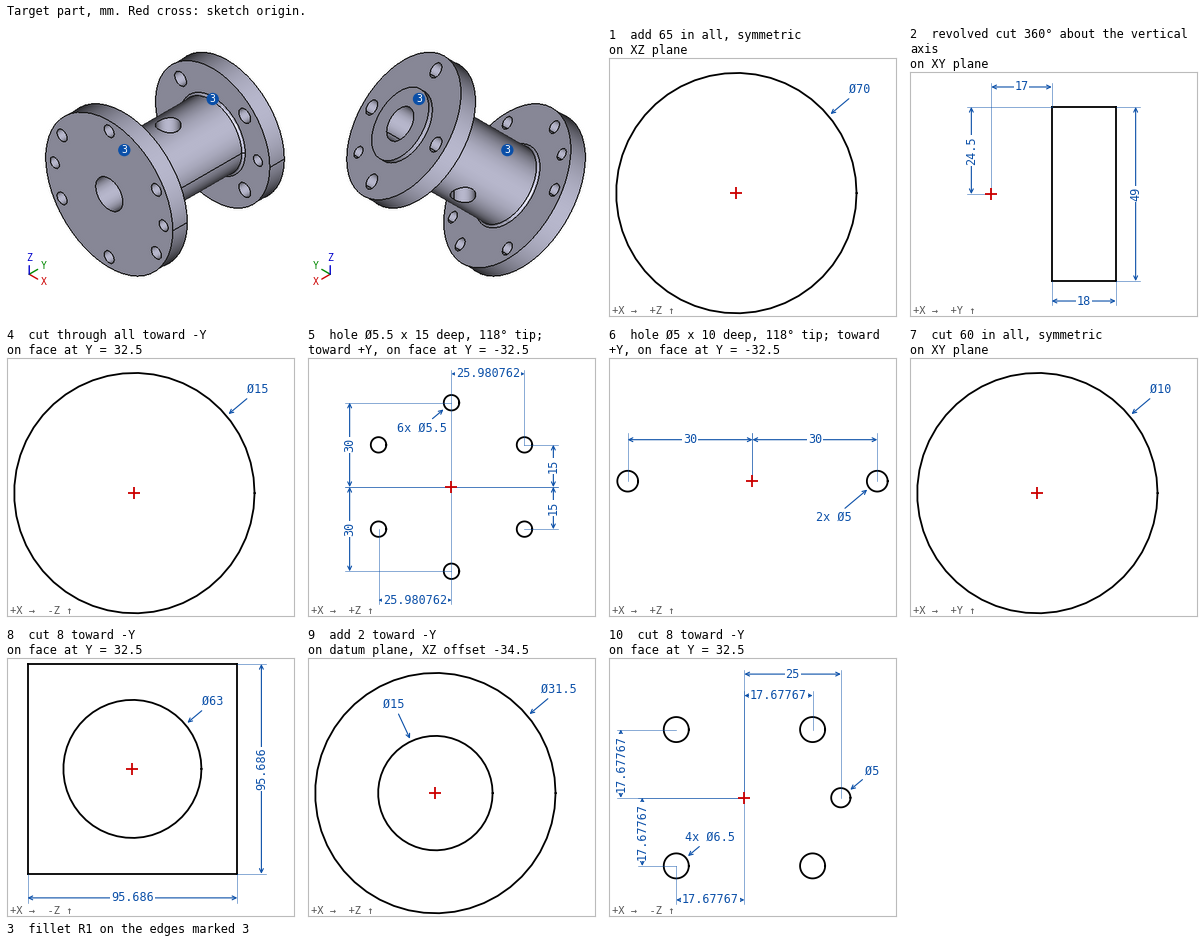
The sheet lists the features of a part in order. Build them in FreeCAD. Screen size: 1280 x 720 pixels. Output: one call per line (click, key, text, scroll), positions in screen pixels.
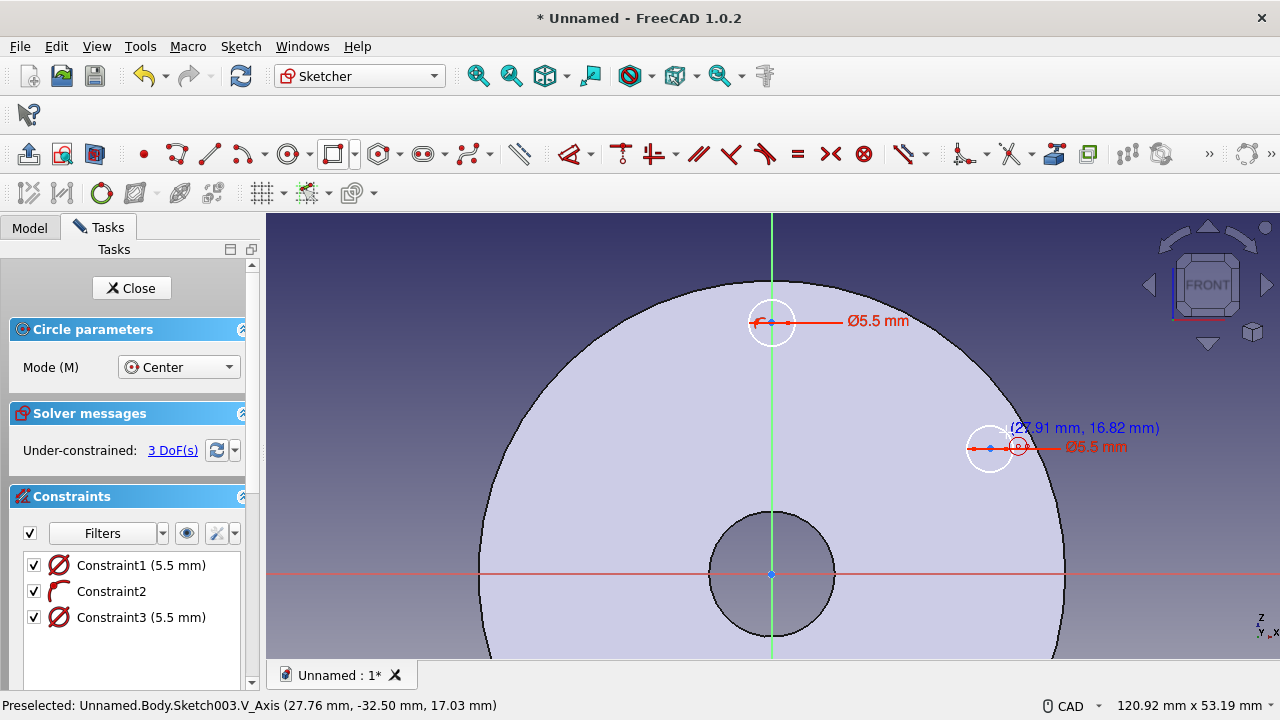
scroll(622, 268, down, 3)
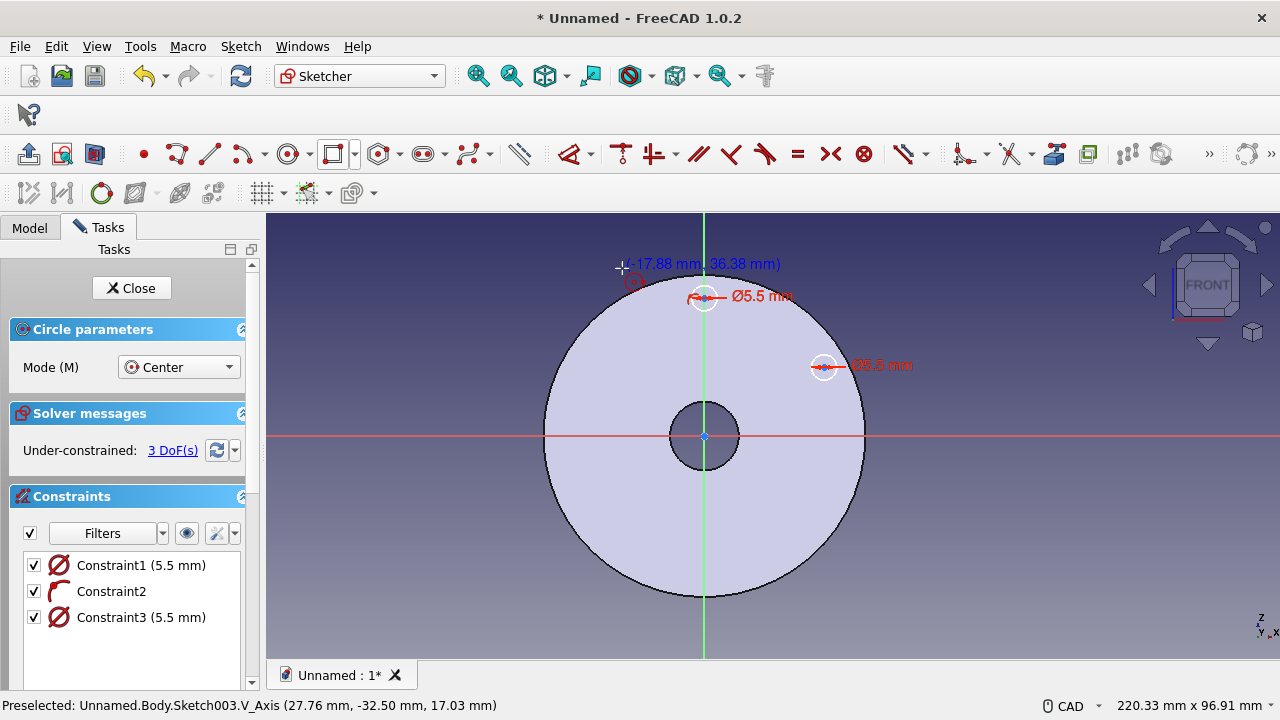
scroll(824, 505, up, 3)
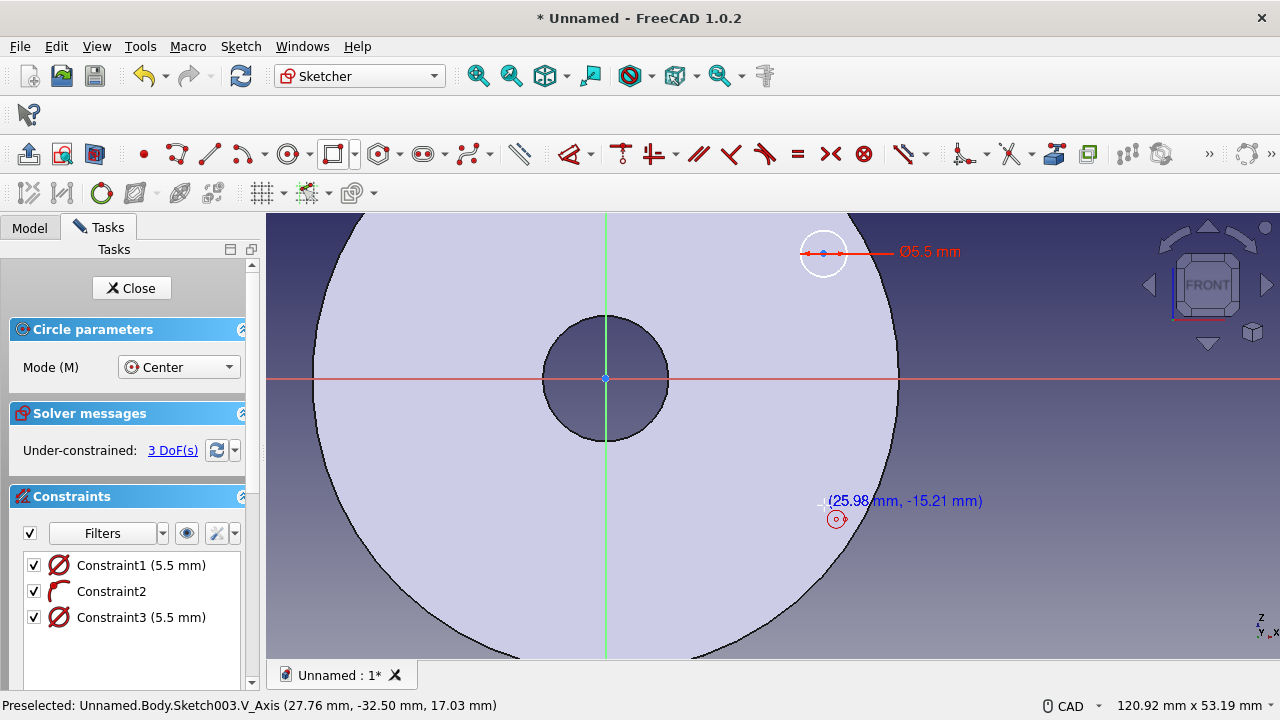
click(824, 505)
move(840, 488)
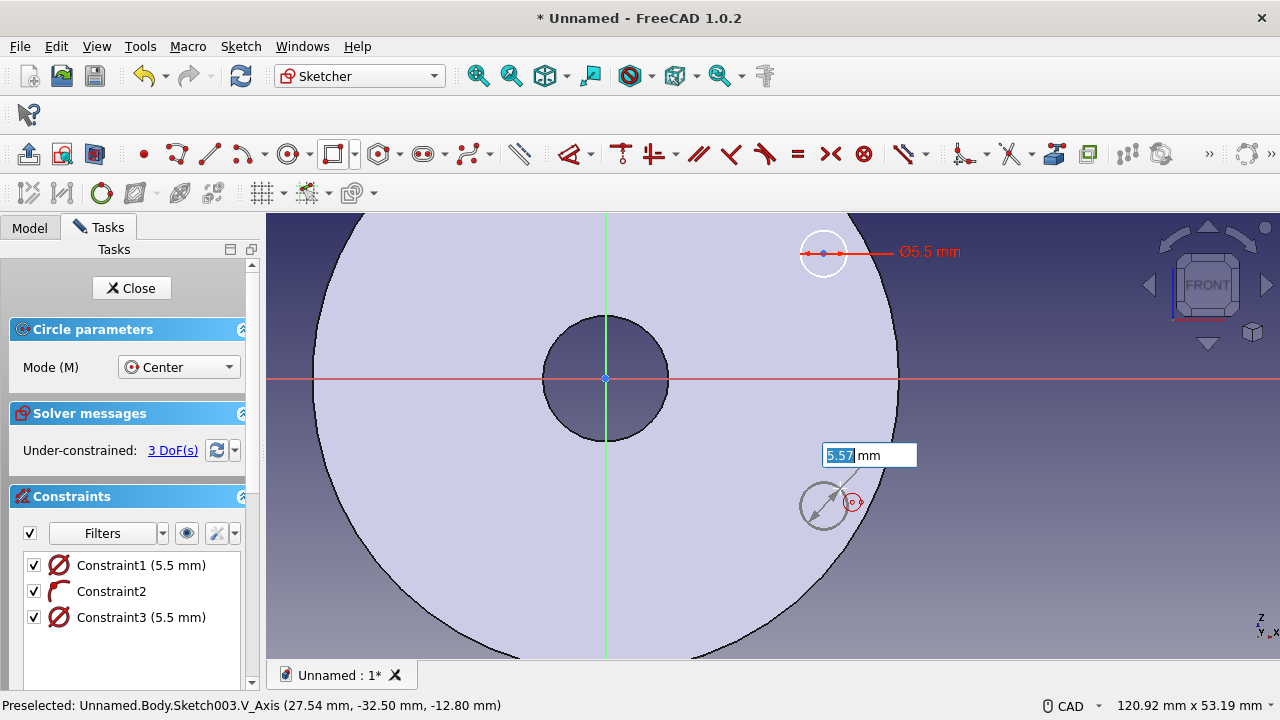
text(5.5)
key(Return)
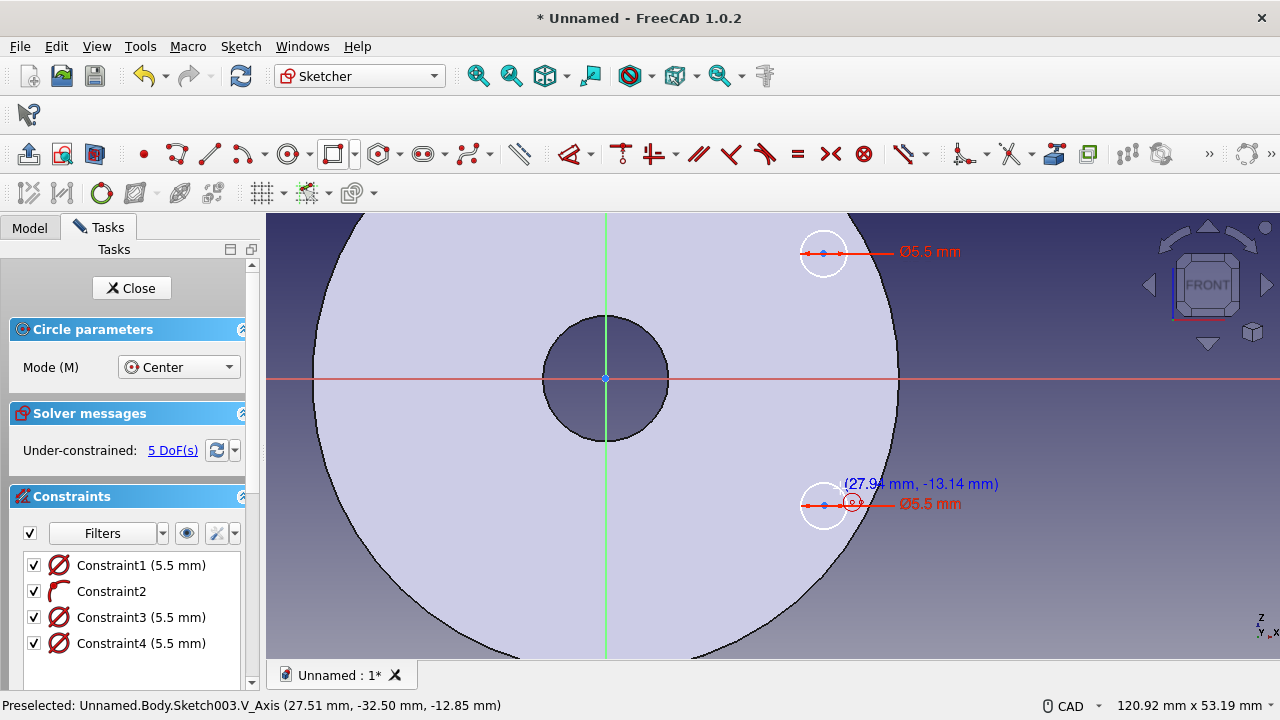
click(606, 630)
move(622, 614)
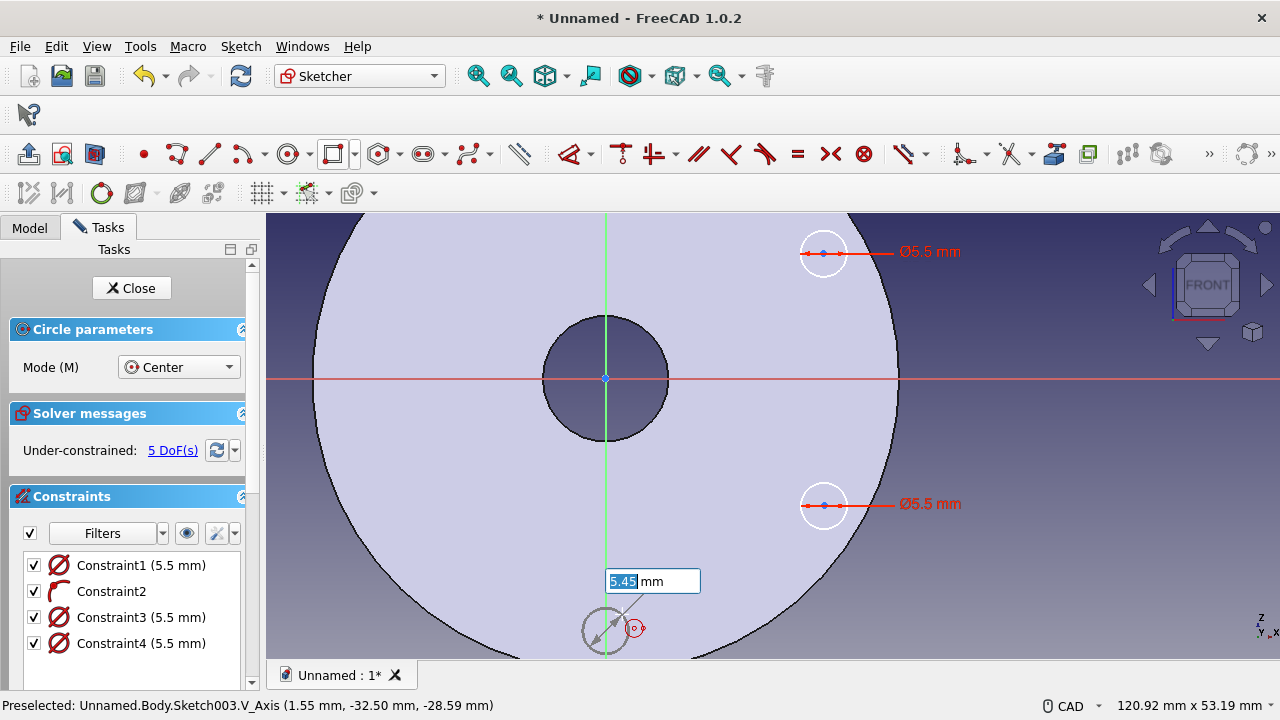
text(5.5)
key(Return)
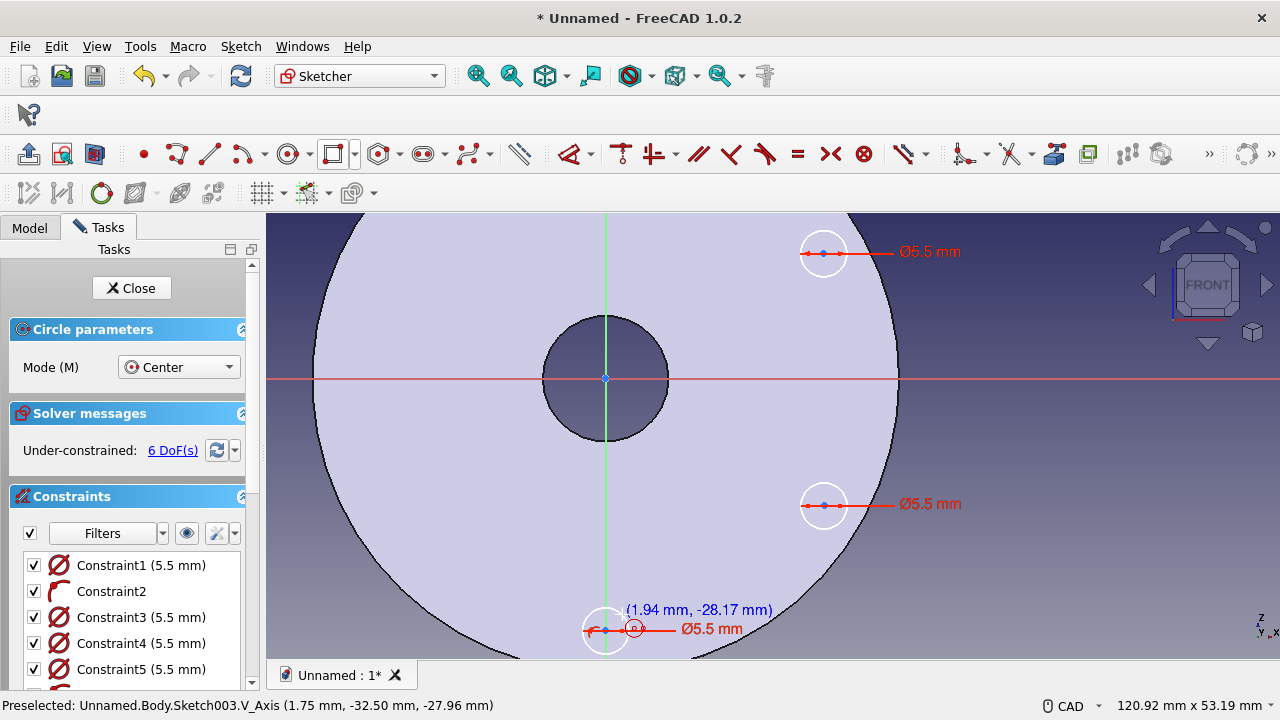
click(388, 505)
move(404, 488)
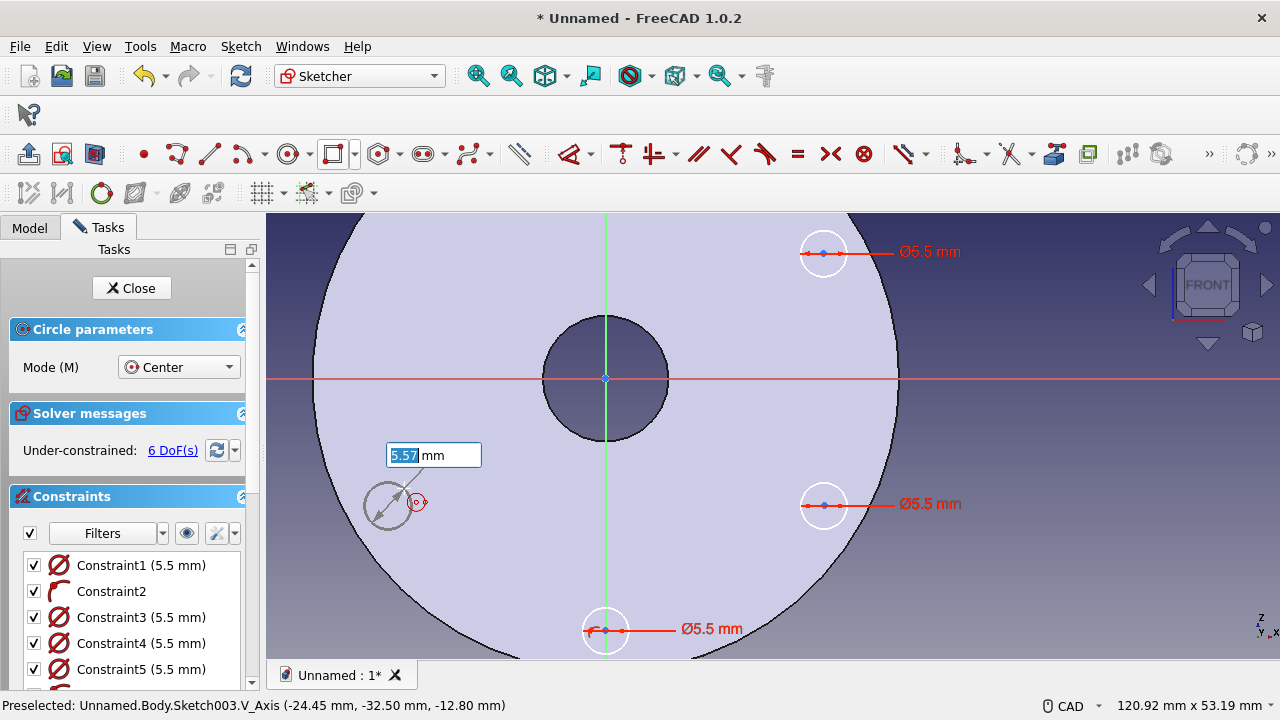
text(5.5)
key(Return)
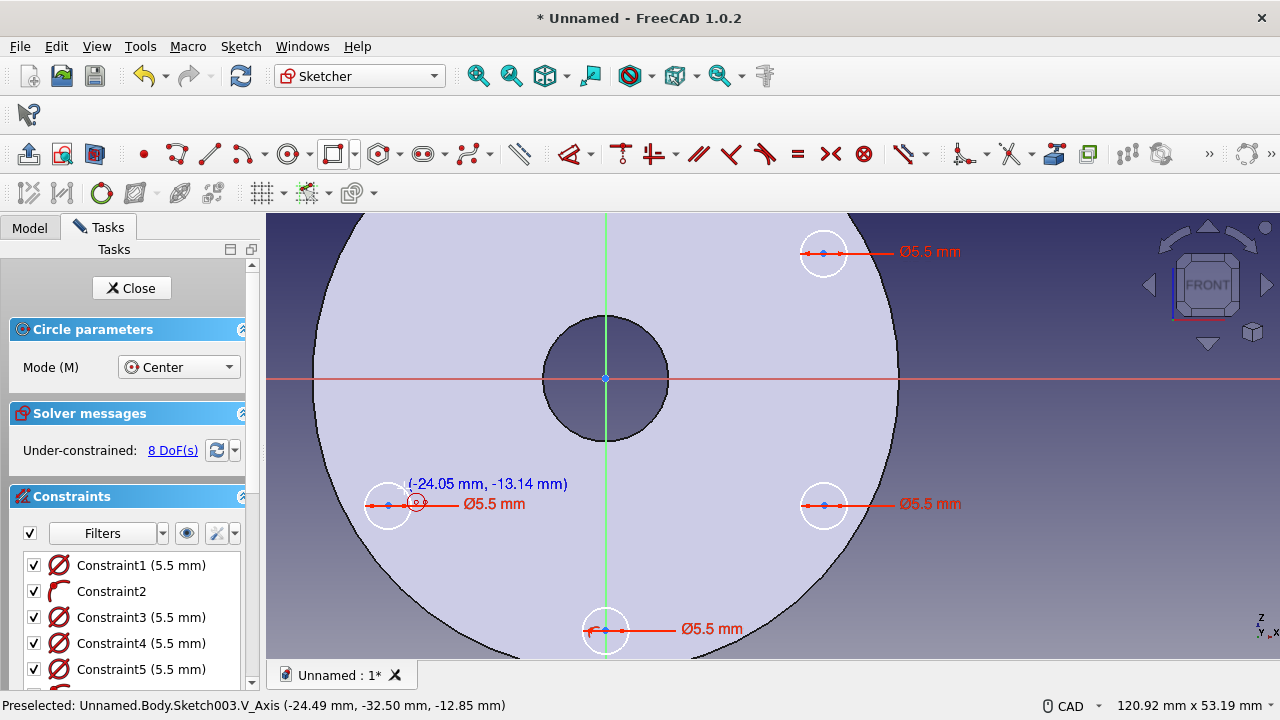
click(388, 253)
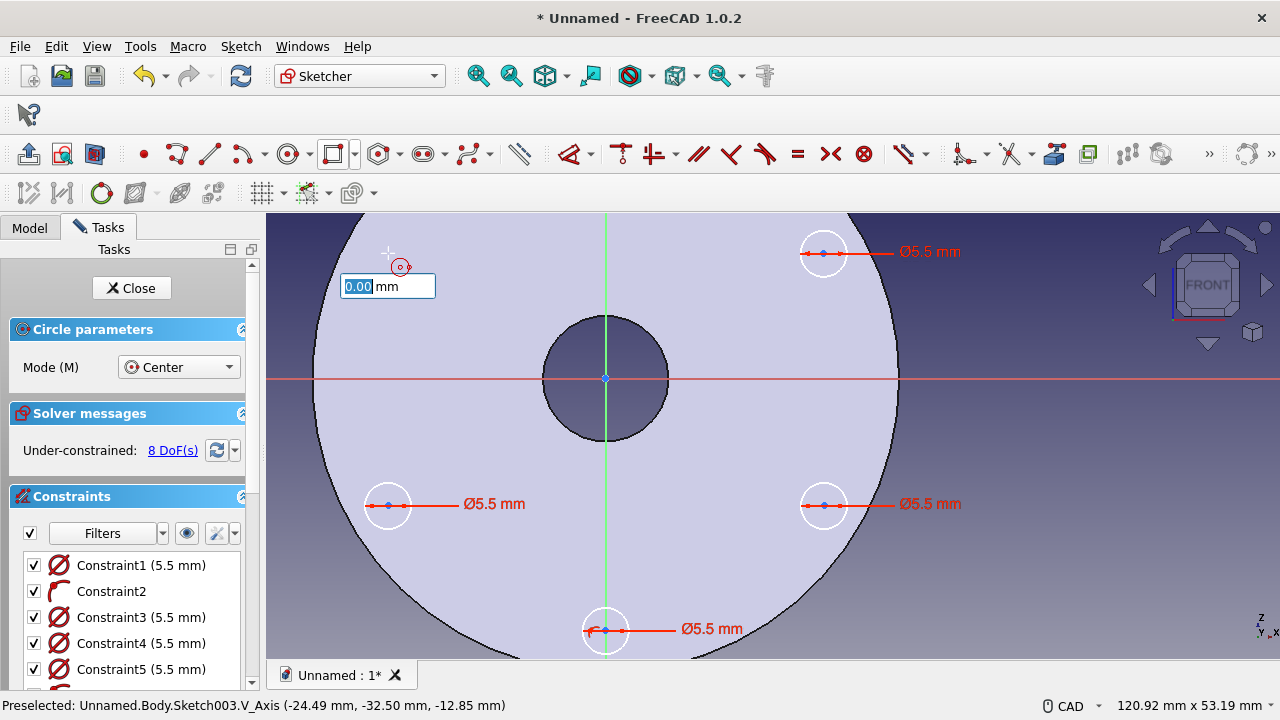
scroll(825, 506, down, 3)
move(594, 358)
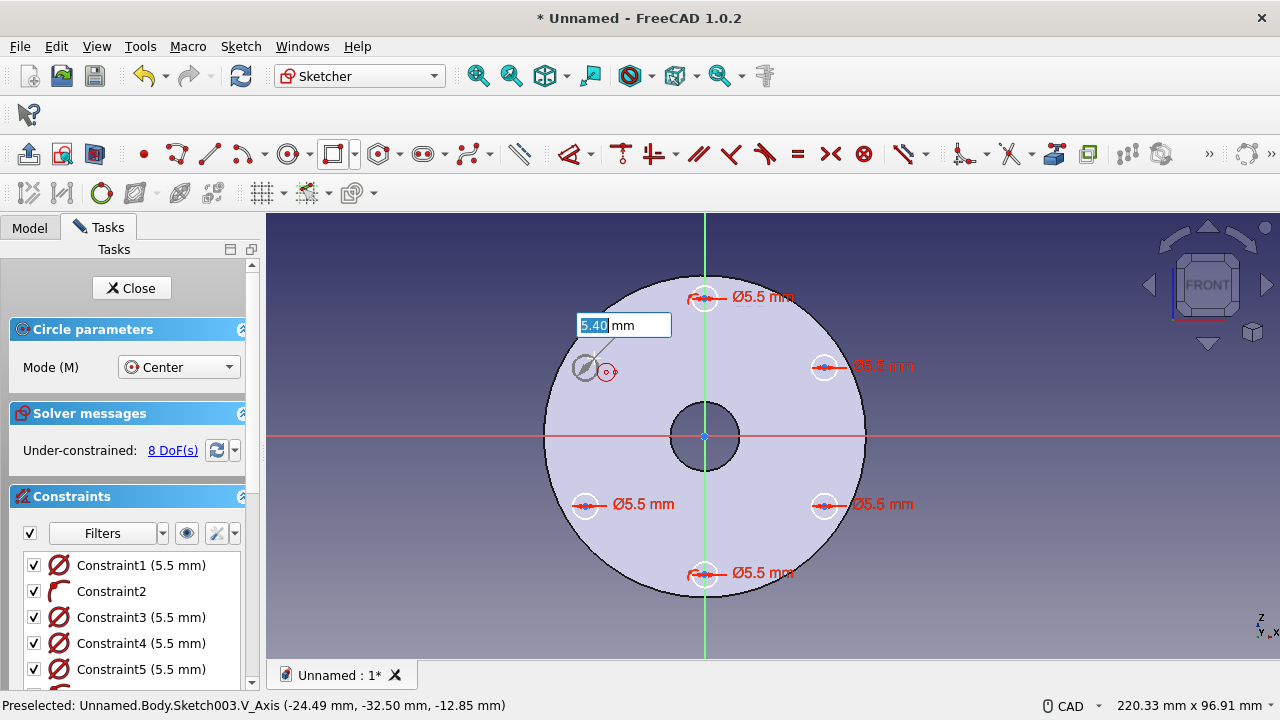
text(5.5)
key(Return)
key(Escape)